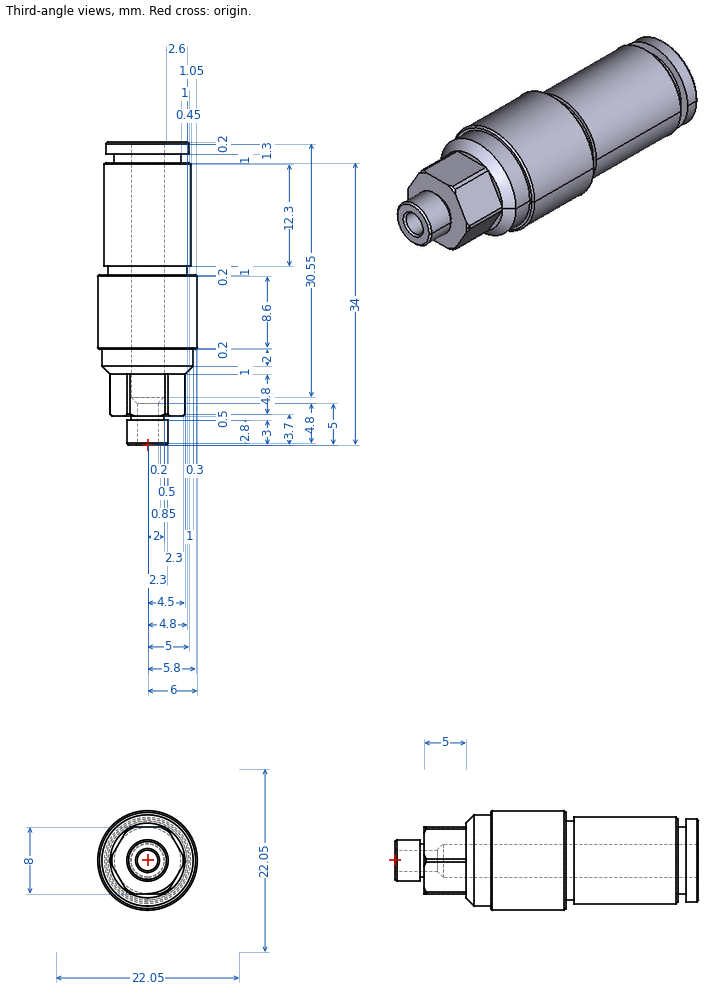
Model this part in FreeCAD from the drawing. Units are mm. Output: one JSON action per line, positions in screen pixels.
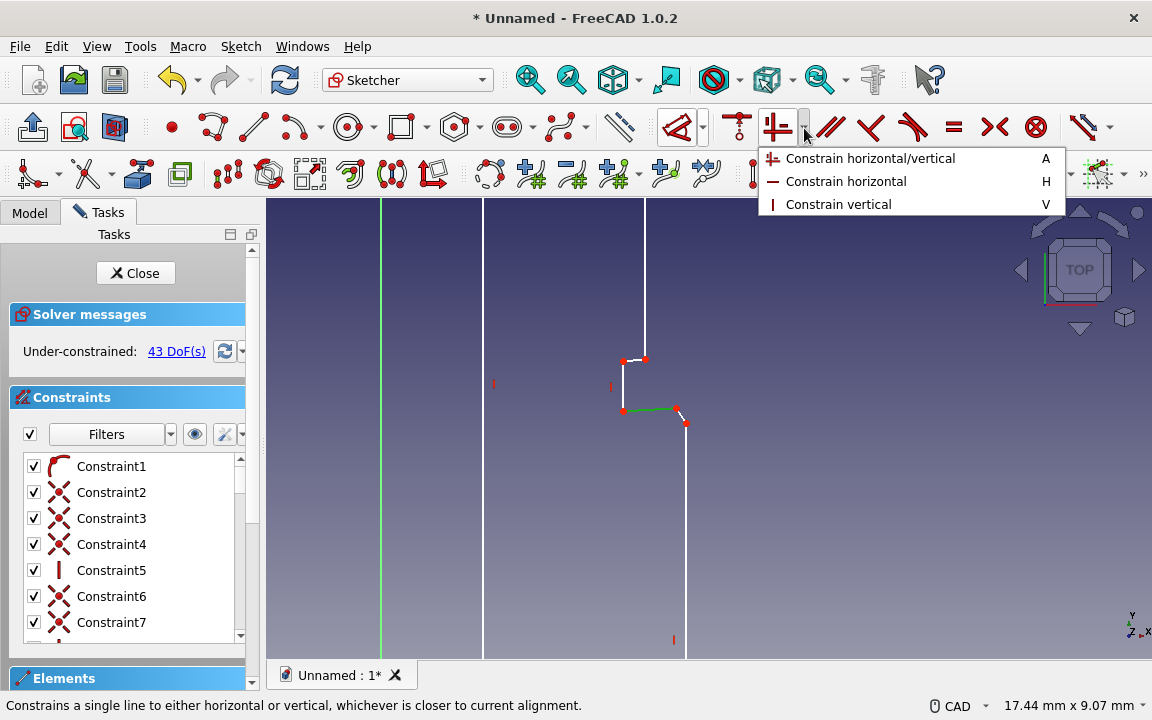
{"action": "left_click", "coordinate": [912, 182]}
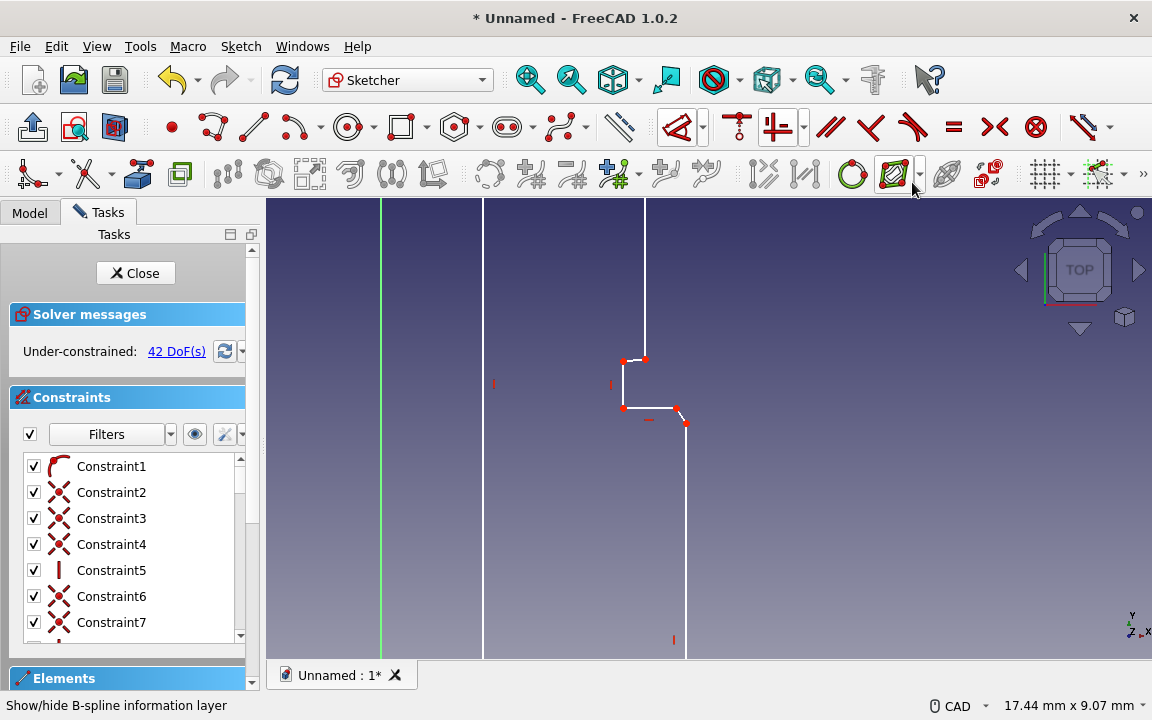
{"action": "scroll", "coordinate": [634, 360], "scroll_direction": "up", "scroll_amount": 2}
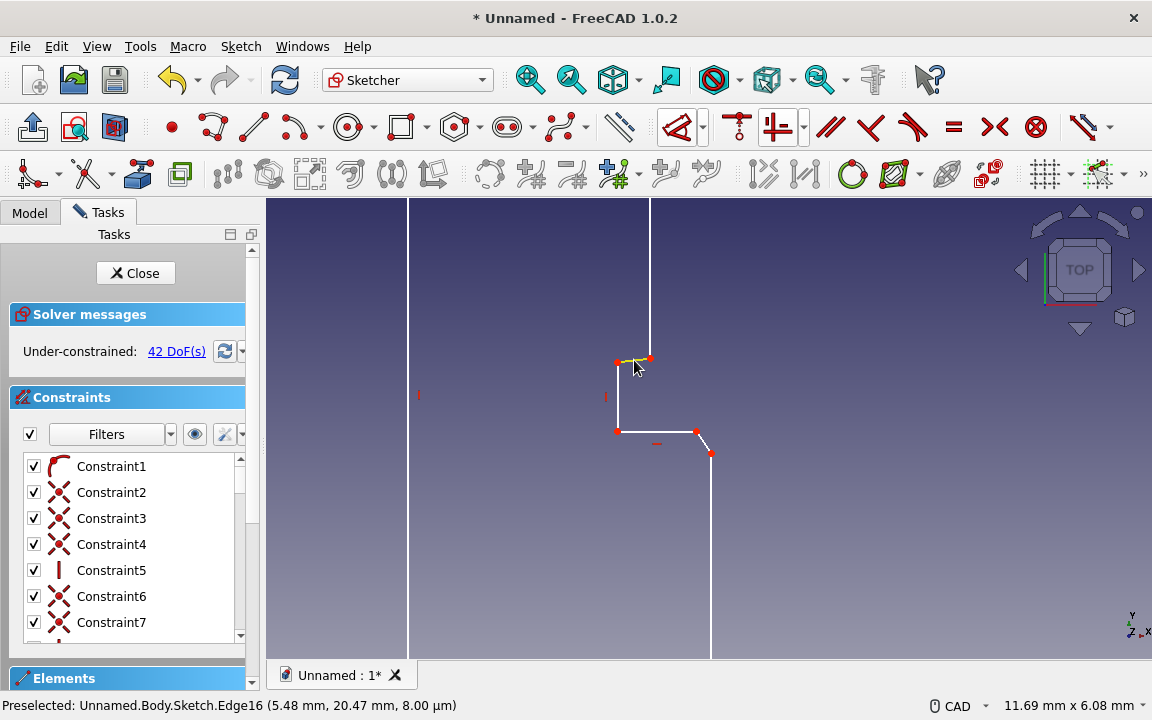
{"action": "left_click", "coordinate": [634, 360]}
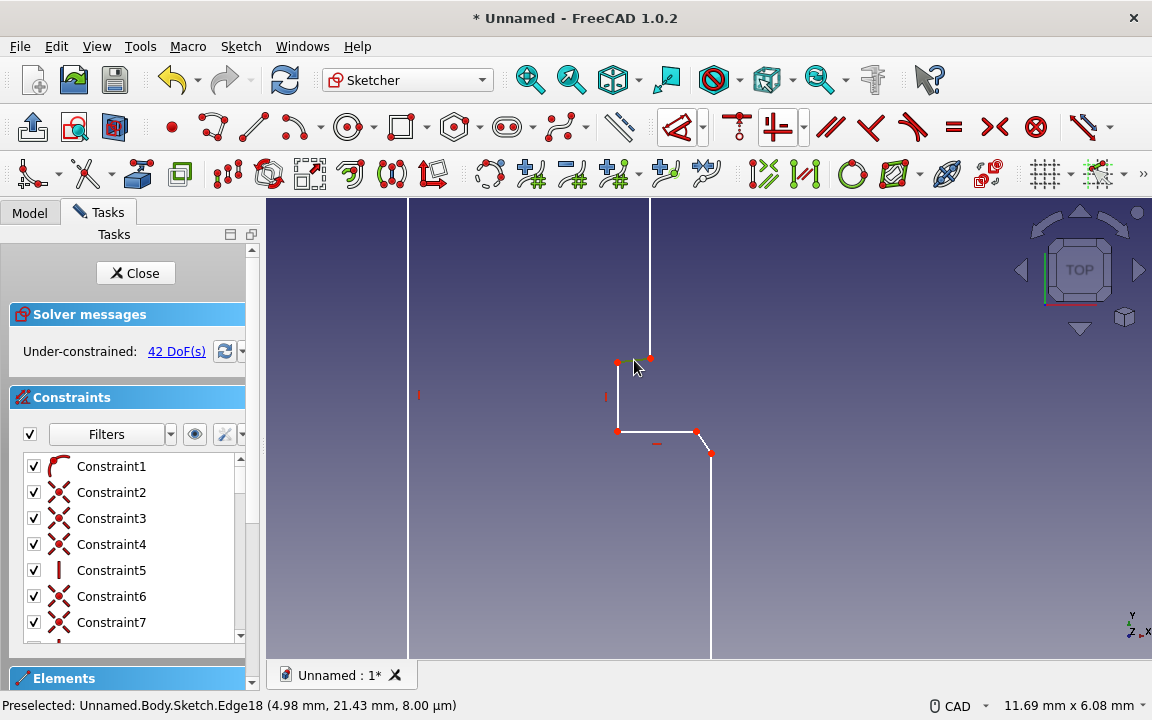
{"action": "left_click", "coordinate": [804, 128]}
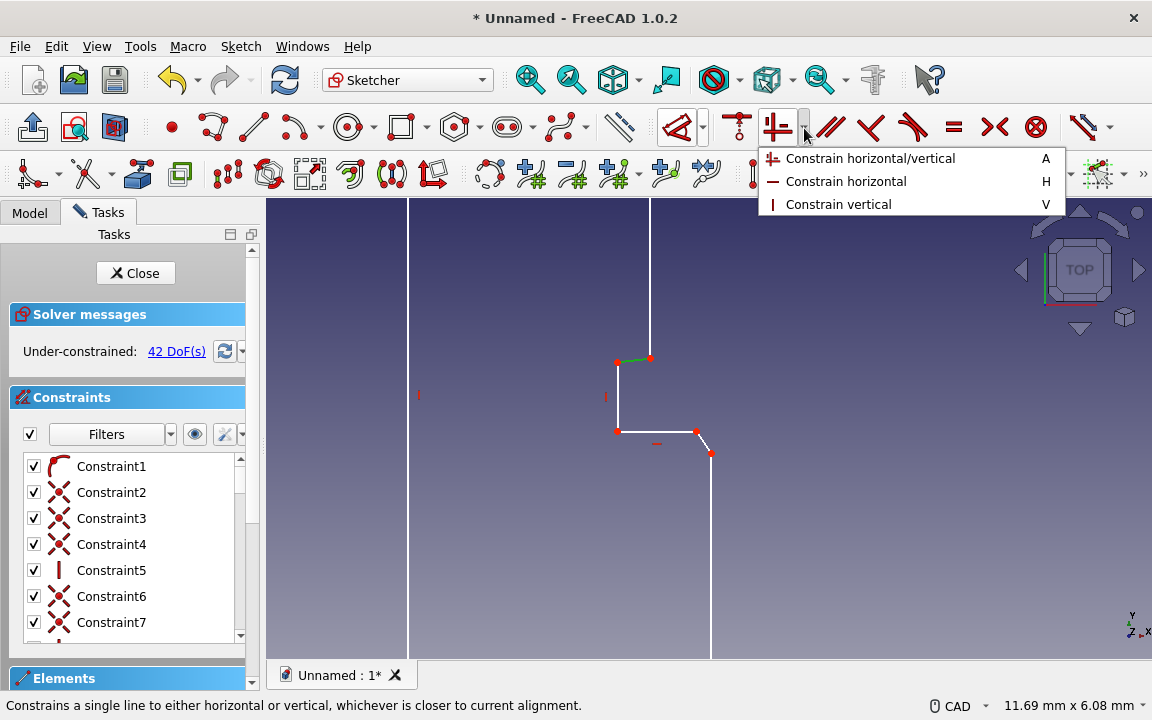
{"action": "left_click", "coordinate": [912, 182]}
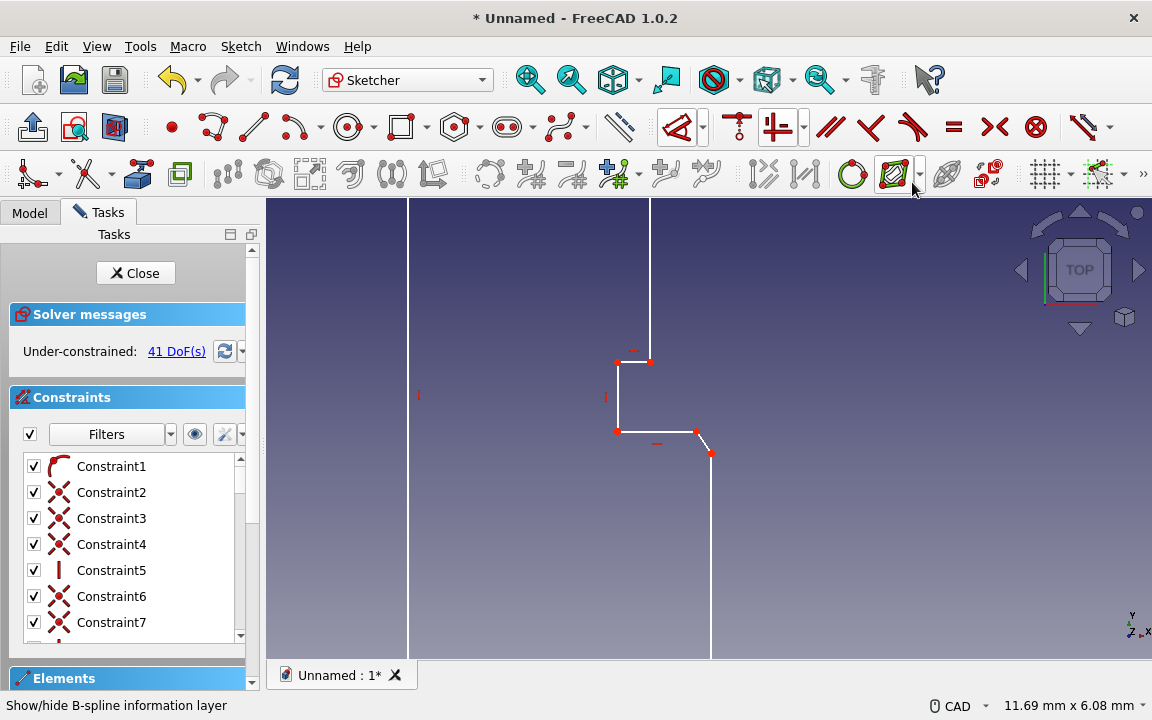
{"action": "scroll", "coordinate": [660, 407], "scroll_direction": "down", "scroll_amount": 11}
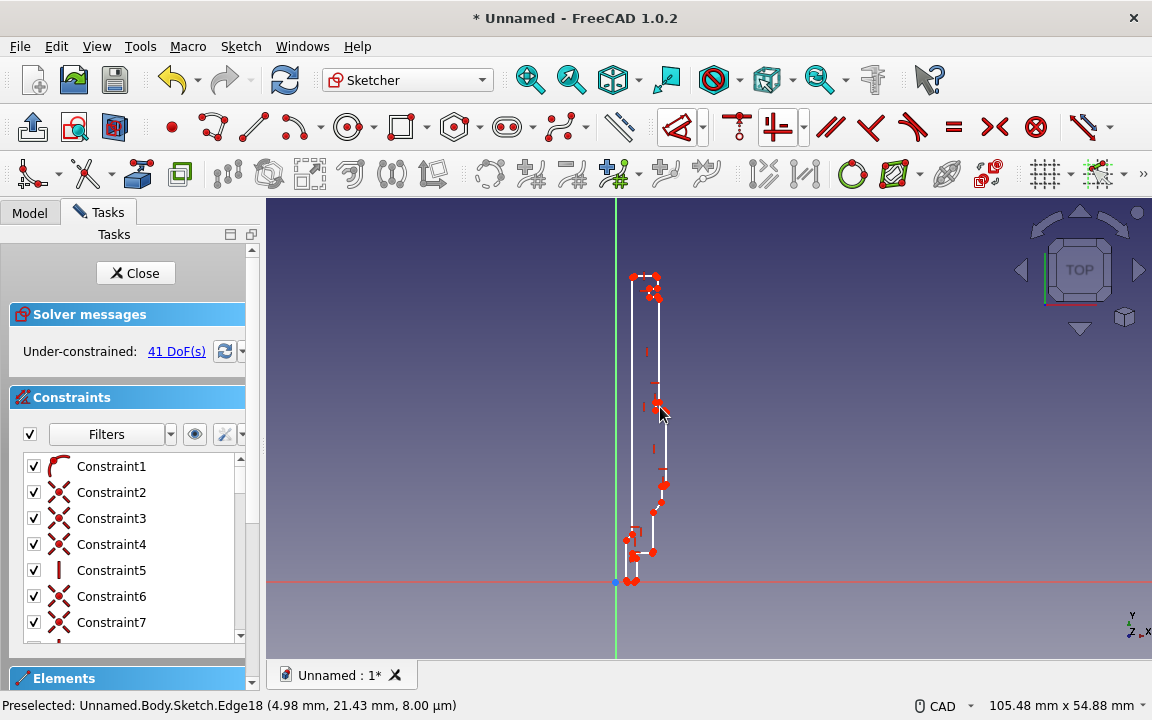
{"action": "scroll", "coordinate": [655, 297], "scroll_direction": "up", "scroll_amount": 9}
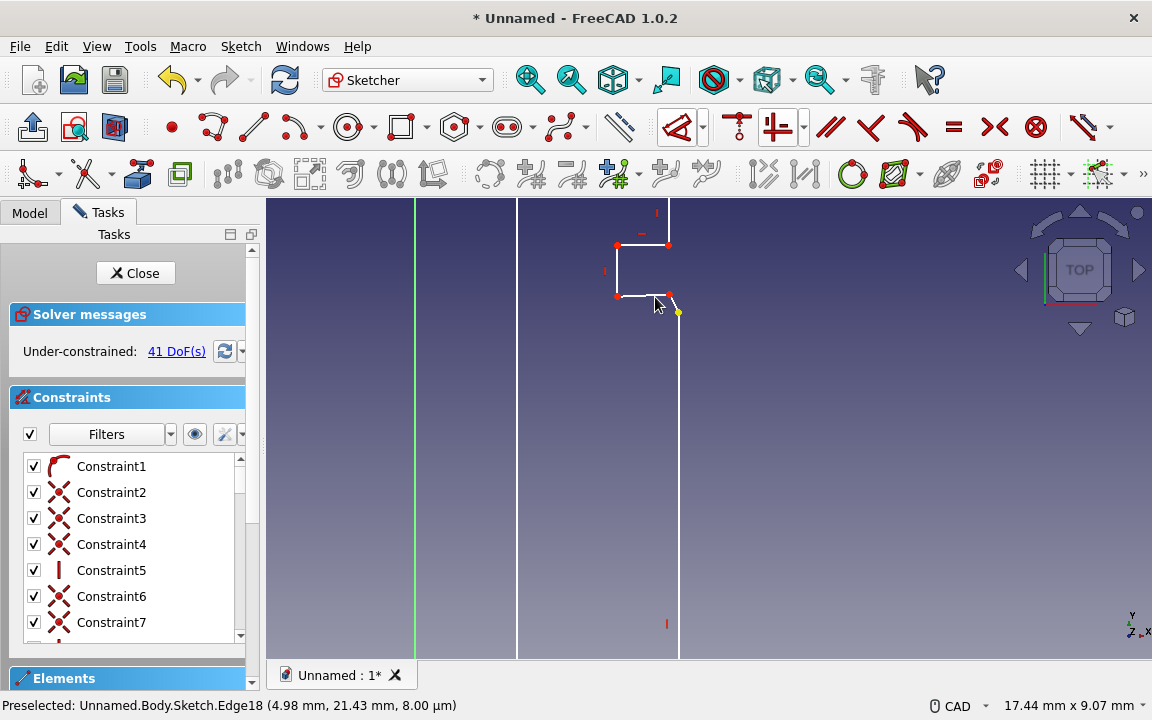
{"action": "left_click", "coordinate": [654, 295]}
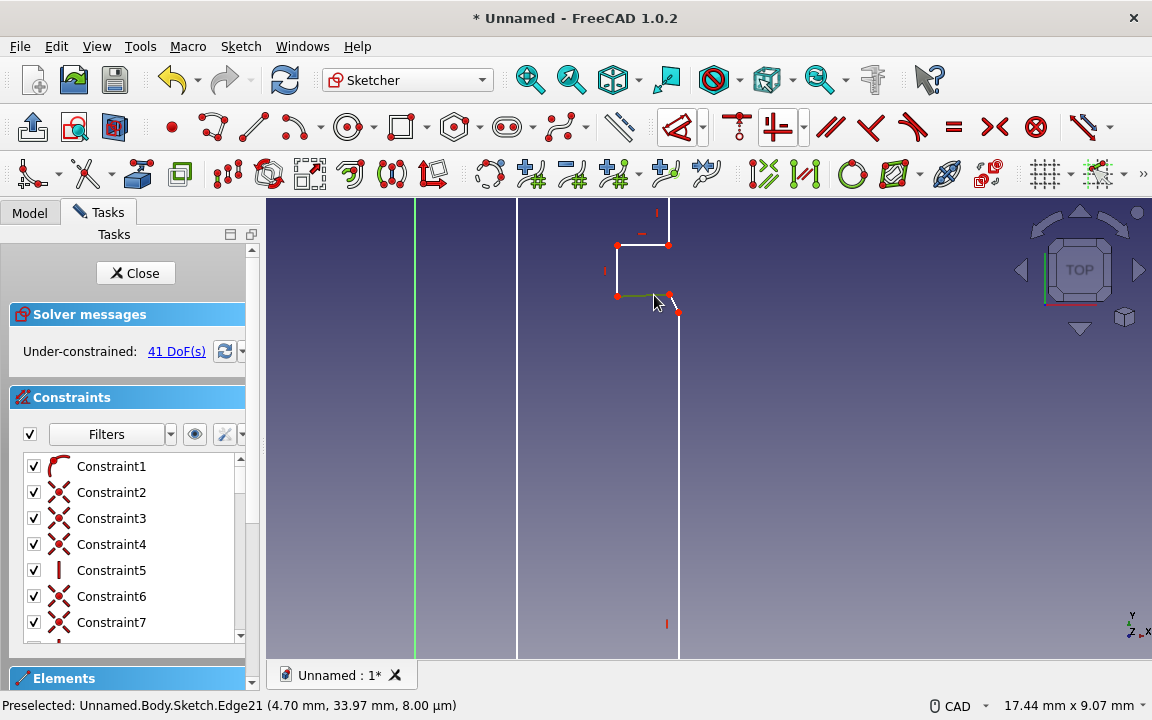
{"action": "left_click", "coordinate": [804, 128]}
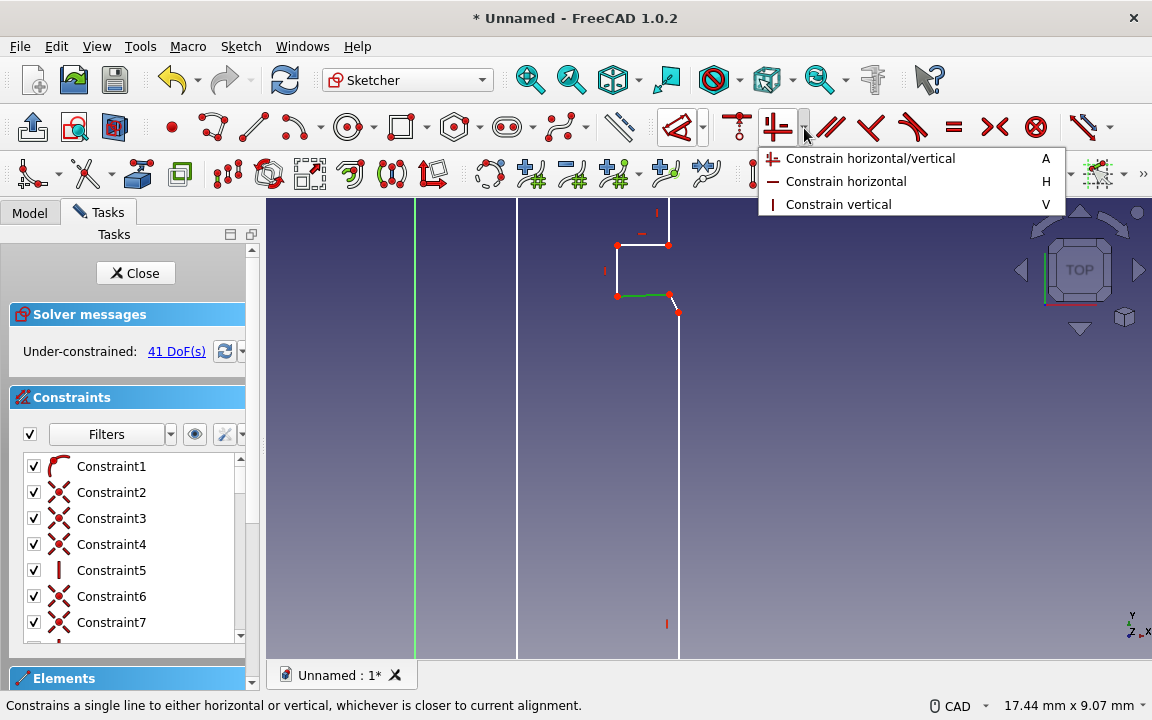
{"action": "left_click", "coordinate": [912, 182]}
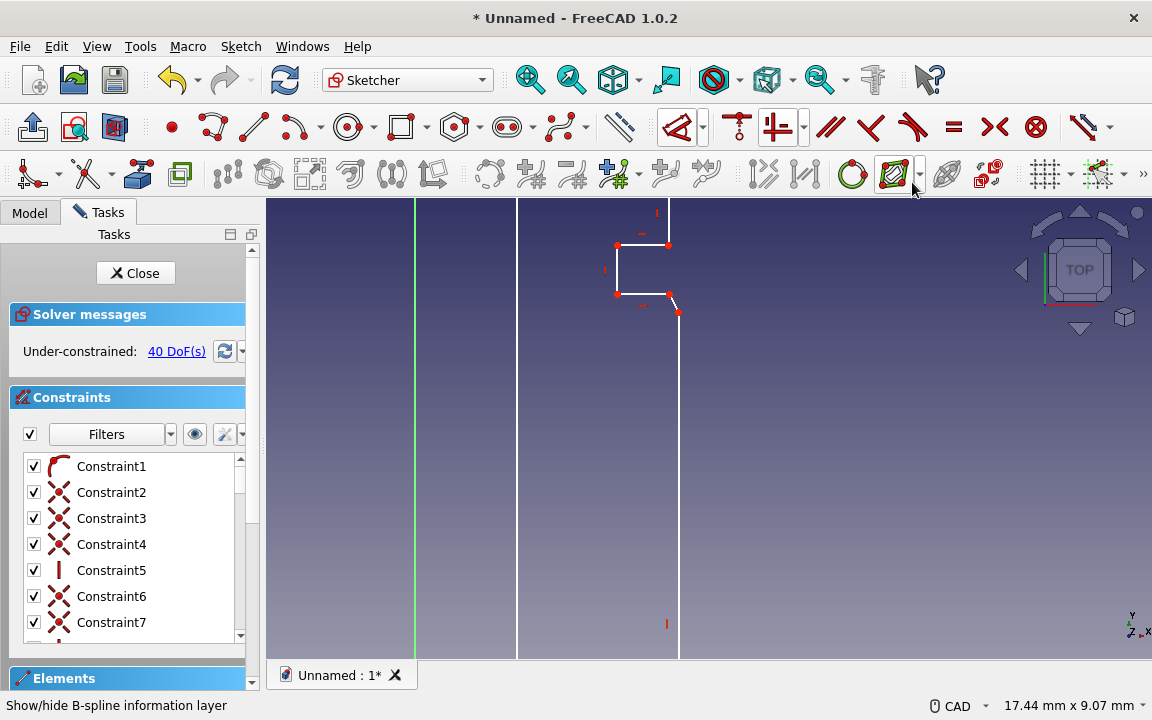
{"action": "scroll", "coordinate": [655, 297], "scroll_direction": "down", "scroll_amount": 9}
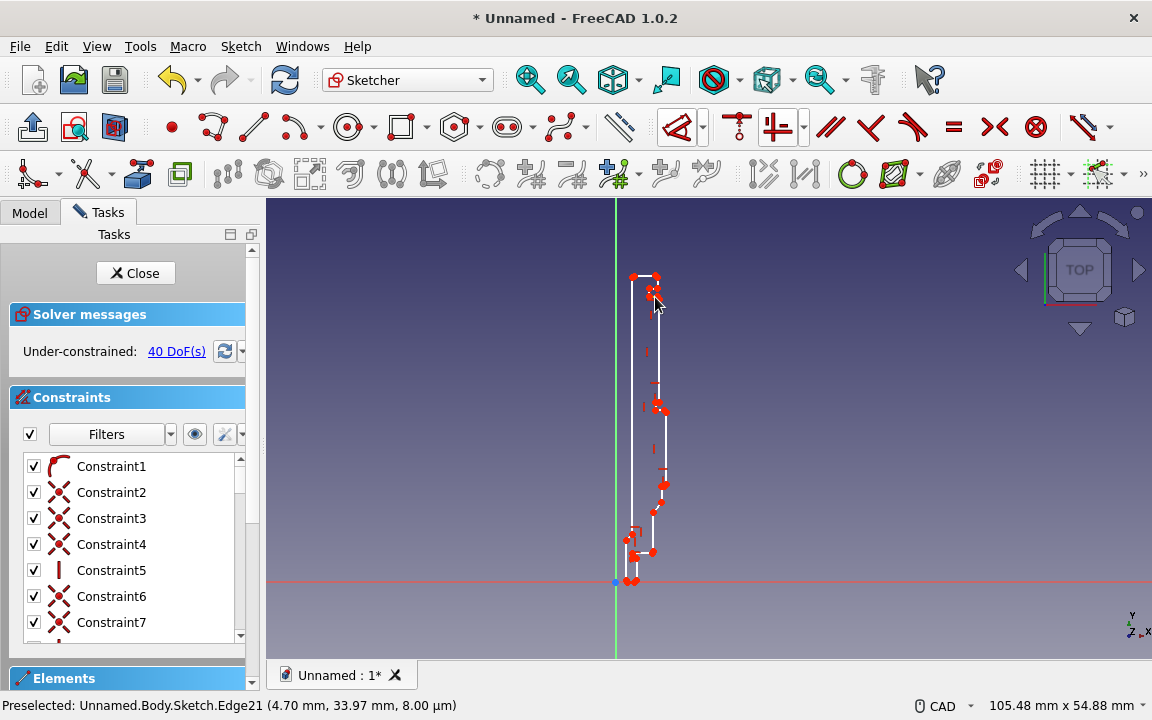
{"action": "scroll", "coordinate": [650, 276], "scroll_direction": "up", "scroll_amount": 4}